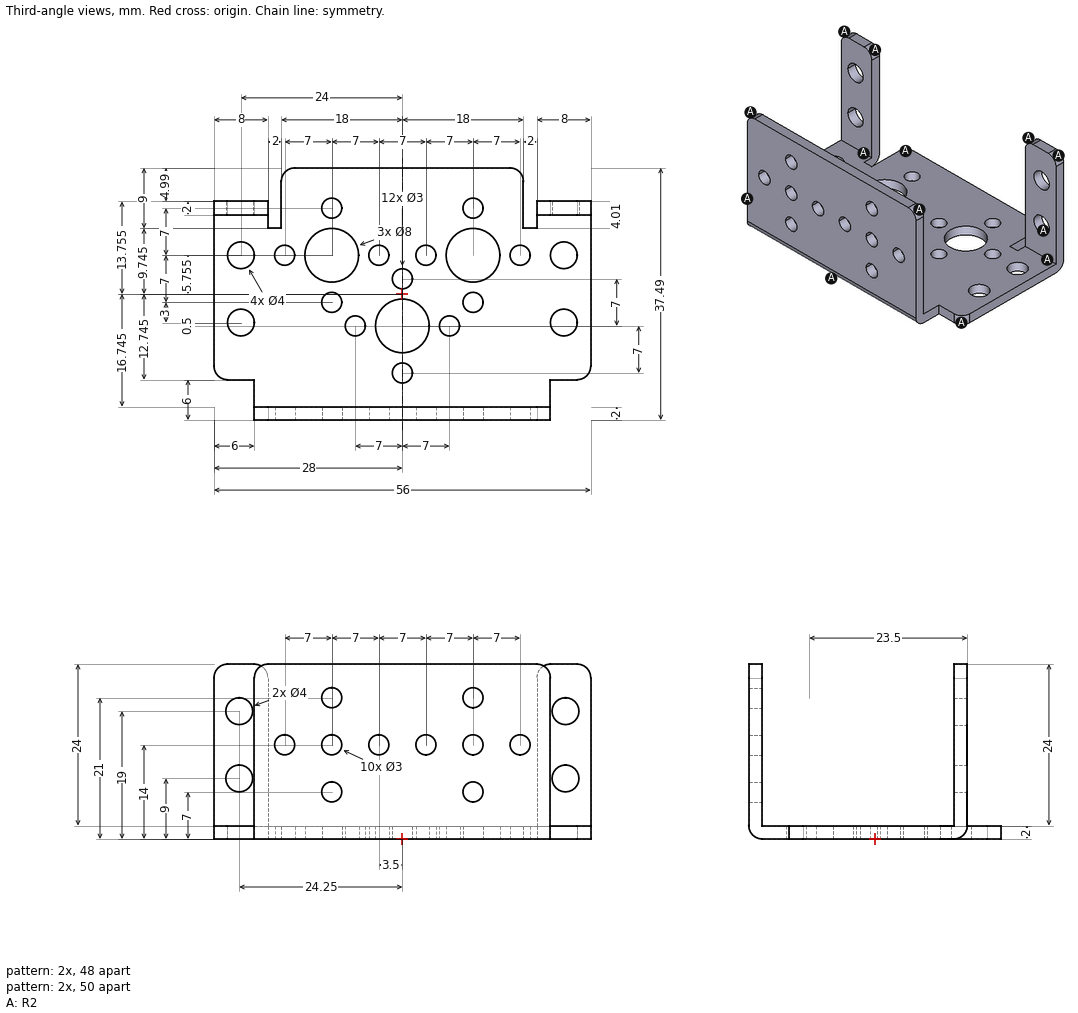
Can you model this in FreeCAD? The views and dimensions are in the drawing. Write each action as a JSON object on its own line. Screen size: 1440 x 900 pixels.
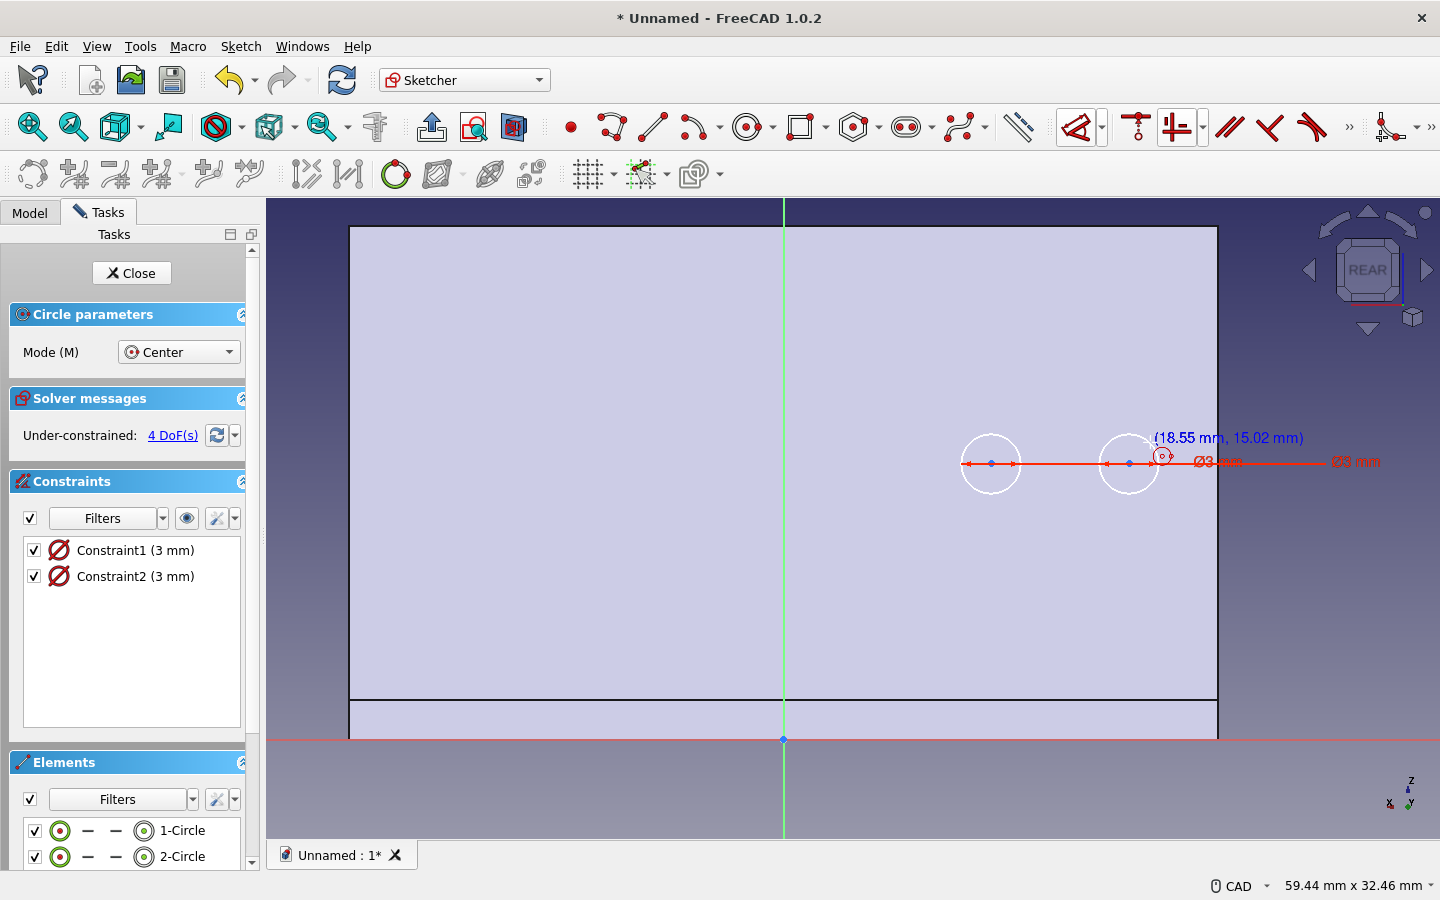
{"action": "left_click", "coordinate": [991, 325]}
{"action": "mouse_move", "coordinate": [1012, 304]}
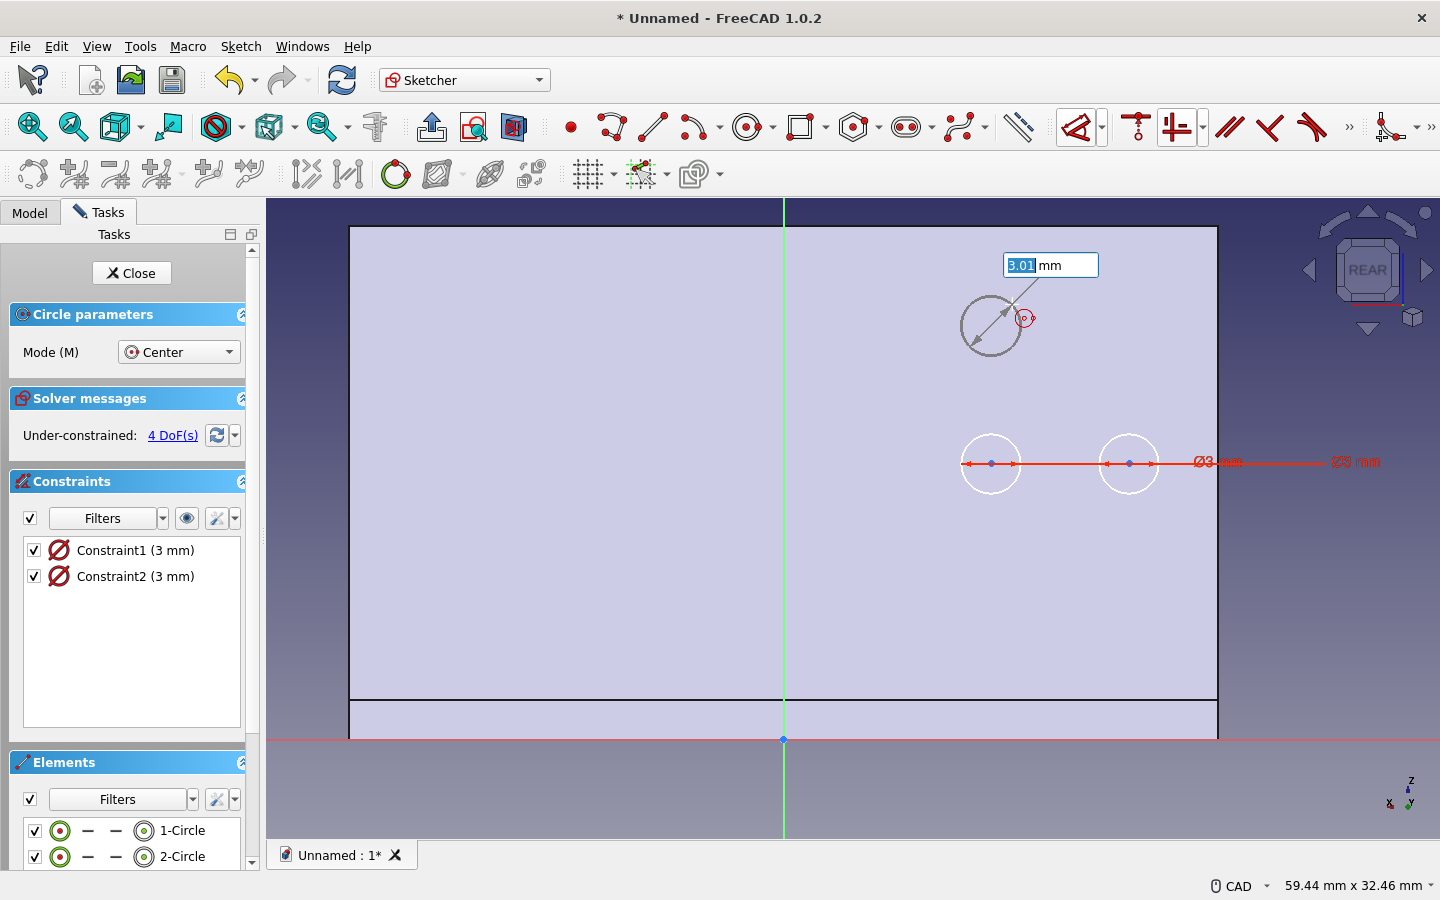
{"action": "type", "text": "3"}
{"action": "key", "text": "Return"}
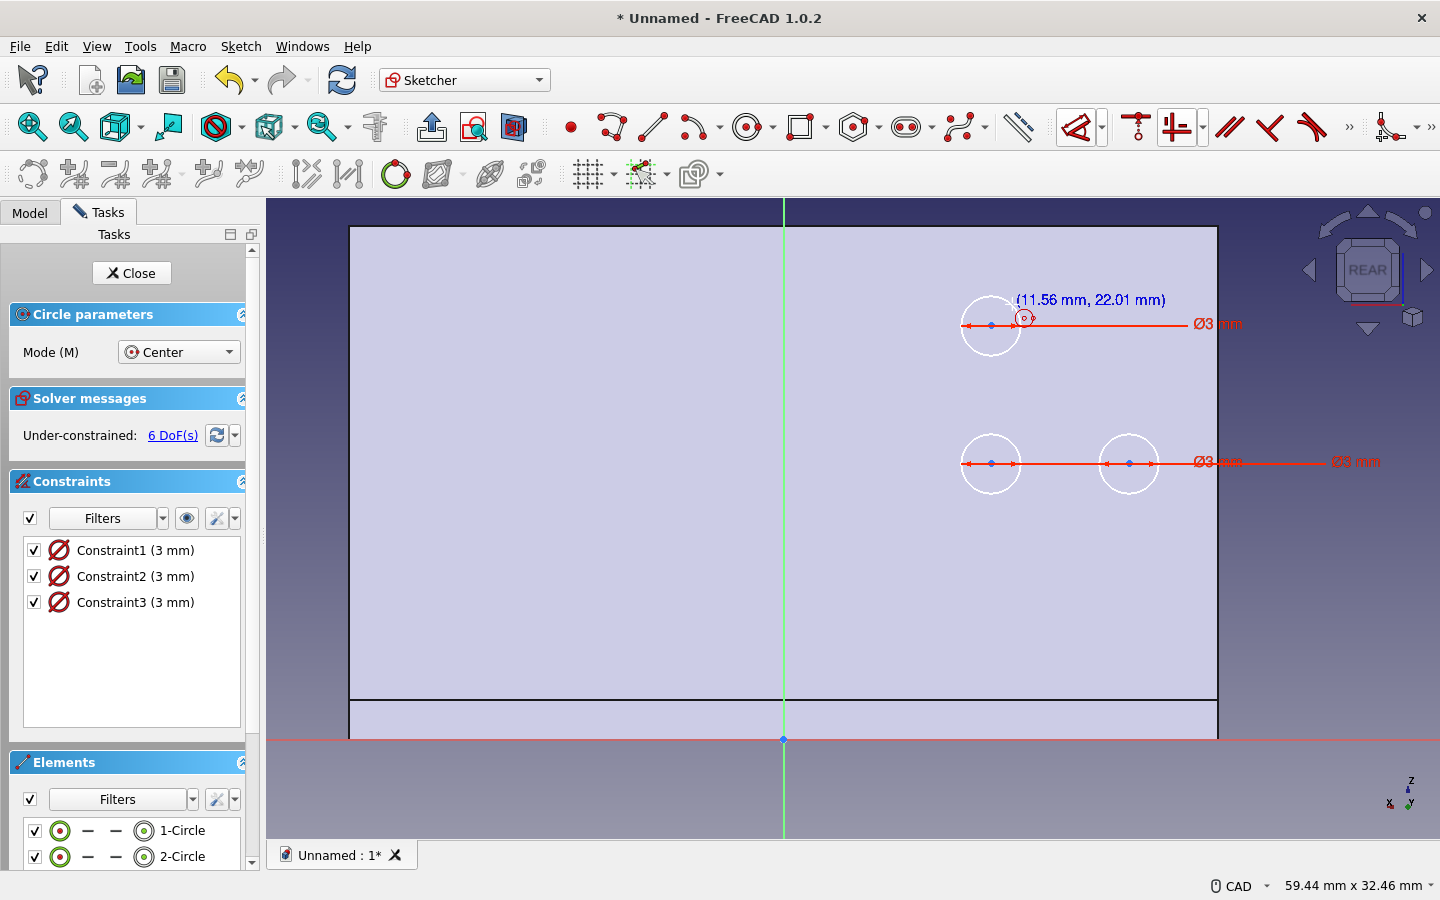
{"action": "left_click", "coordinate": [853, 463]}
{"action": "mouse_move", "coordinate": [874, 442]}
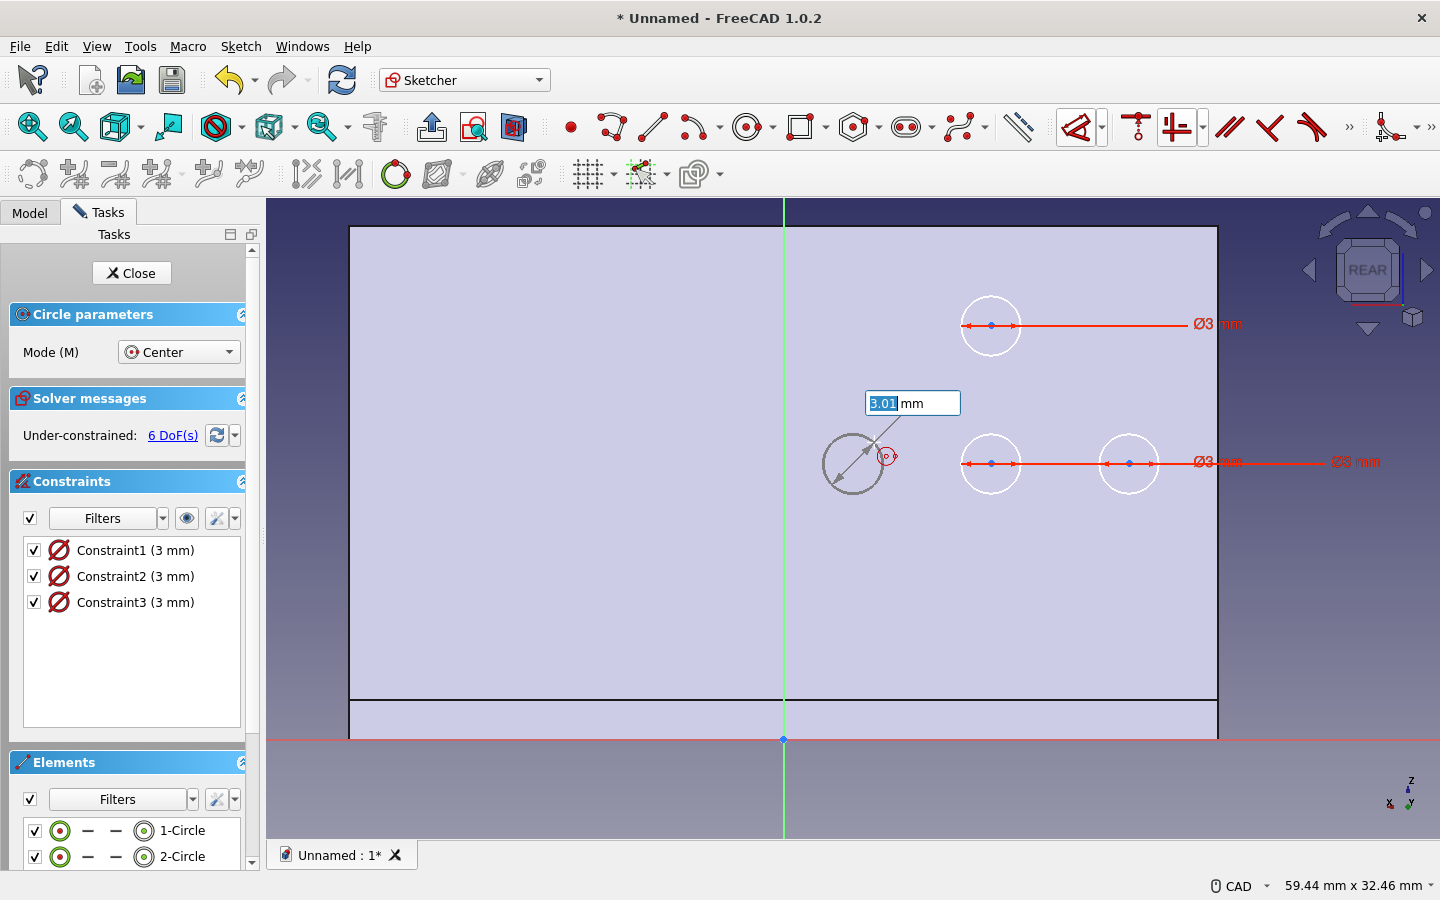
{"action": "type", "text": "3"}
{"action": "key", "text": "Return"}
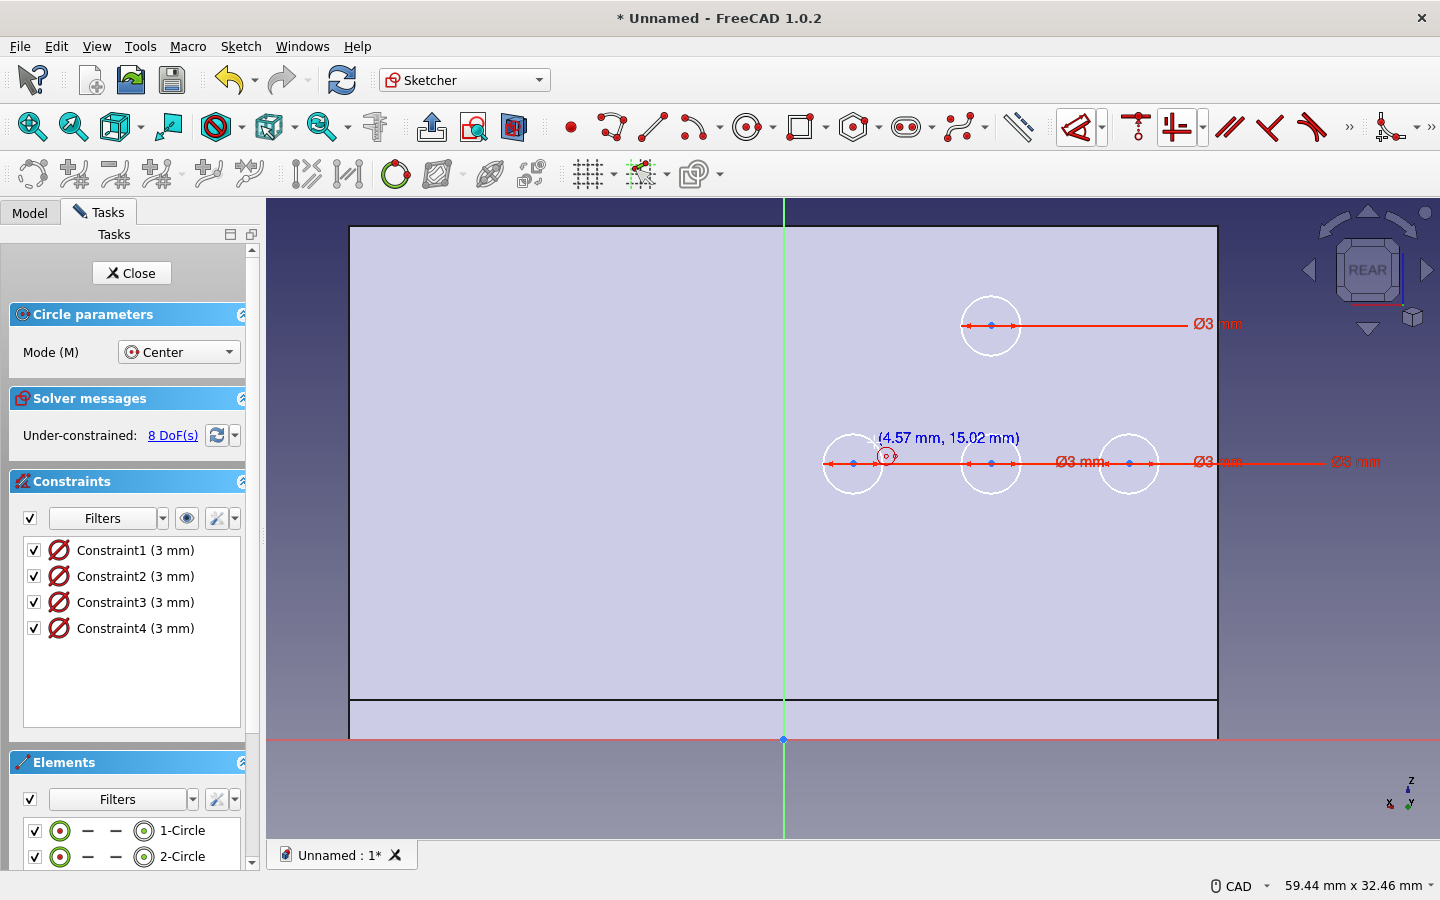
{"action": "left_click", "coordinate": [991, 601]}
{"action": "mouse_move", "coordinate": [1012, 580]}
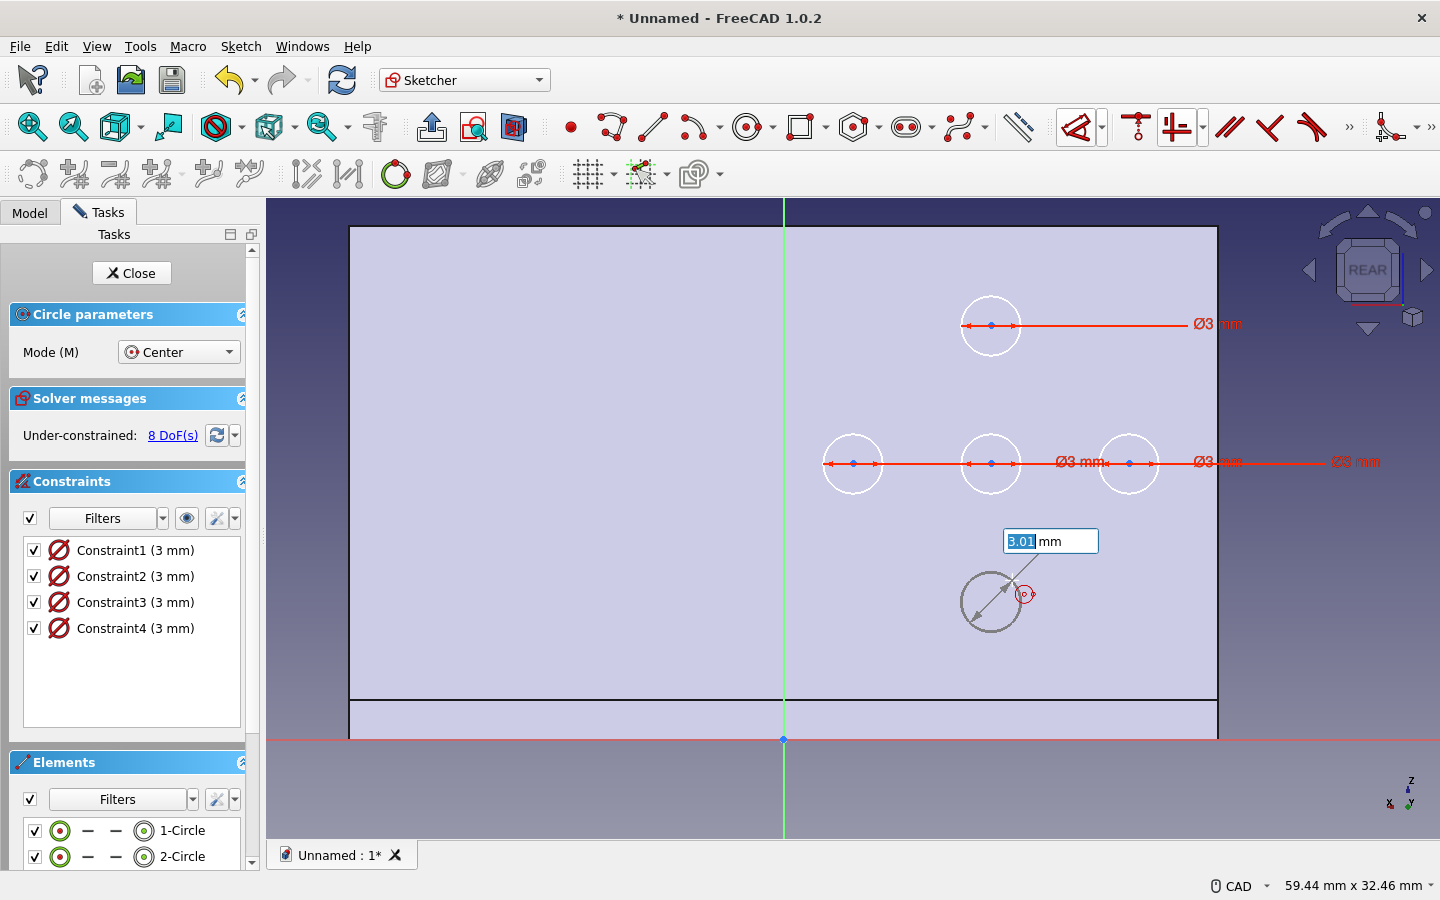
{"action": "type", "text": "3"}
{"action": "key", "text": "Return"}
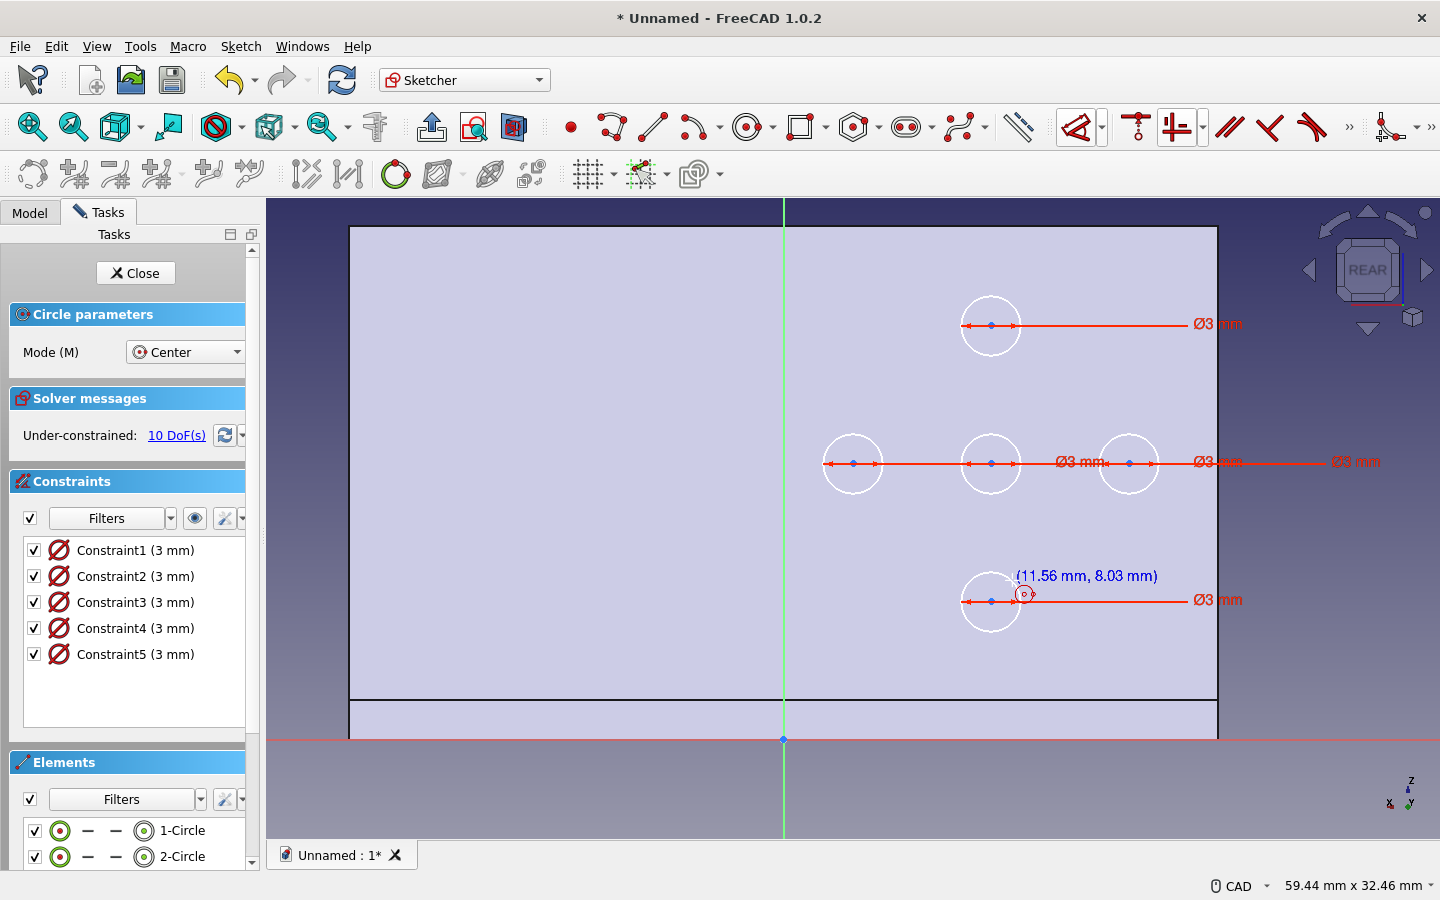
{"action": "left_click", "coordinate": [576, 325]}
{"action": "mouse_move", "coordinate": [597, 304]}